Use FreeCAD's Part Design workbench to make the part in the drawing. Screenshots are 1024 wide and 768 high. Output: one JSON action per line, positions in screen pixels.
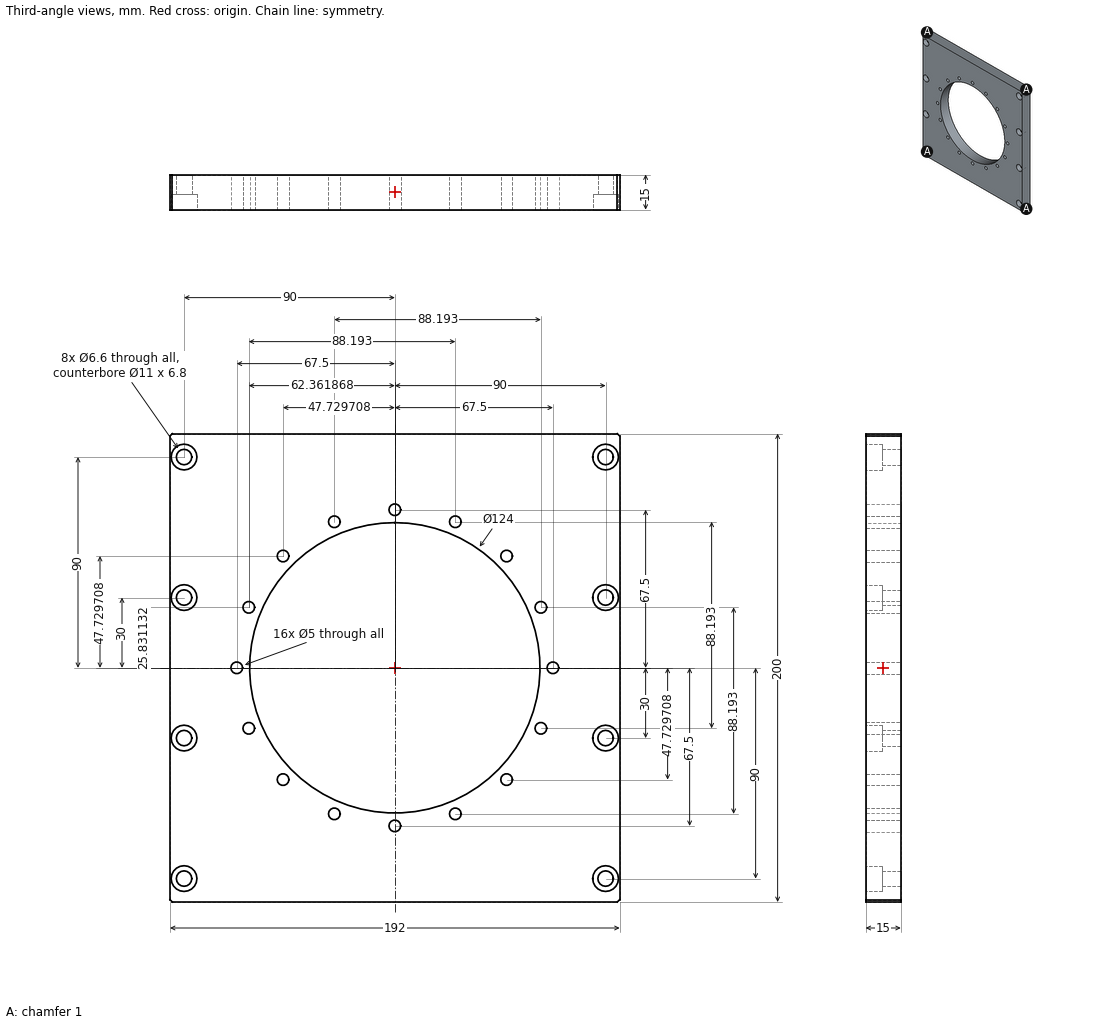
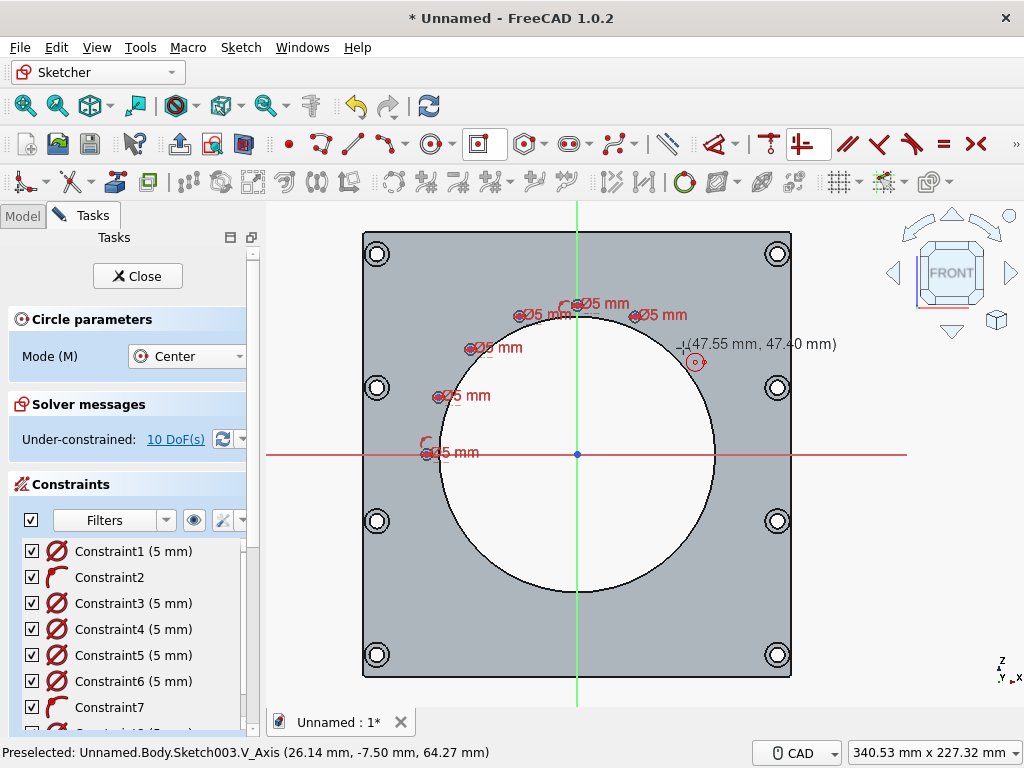
{"action": "left_click", "coordinate": [683, 348]}
{"action": "mouse_move", "coordinate": [687, 344]}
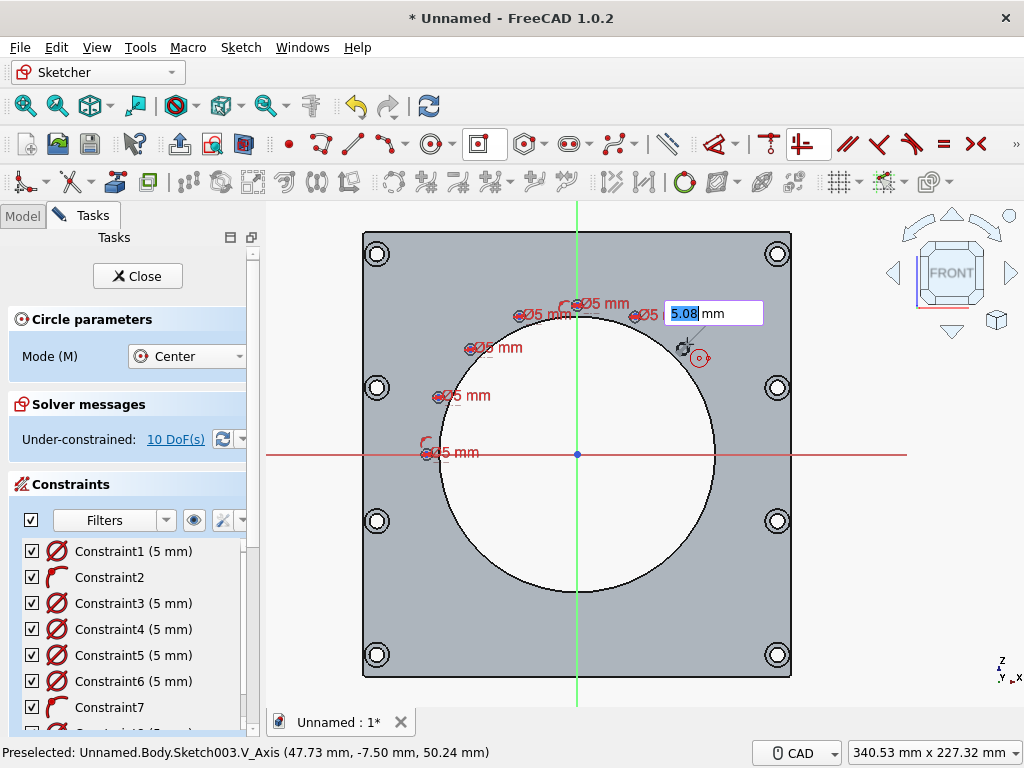
{"action": "type", "text": "5"}
{"action": "key", "text": "Return"}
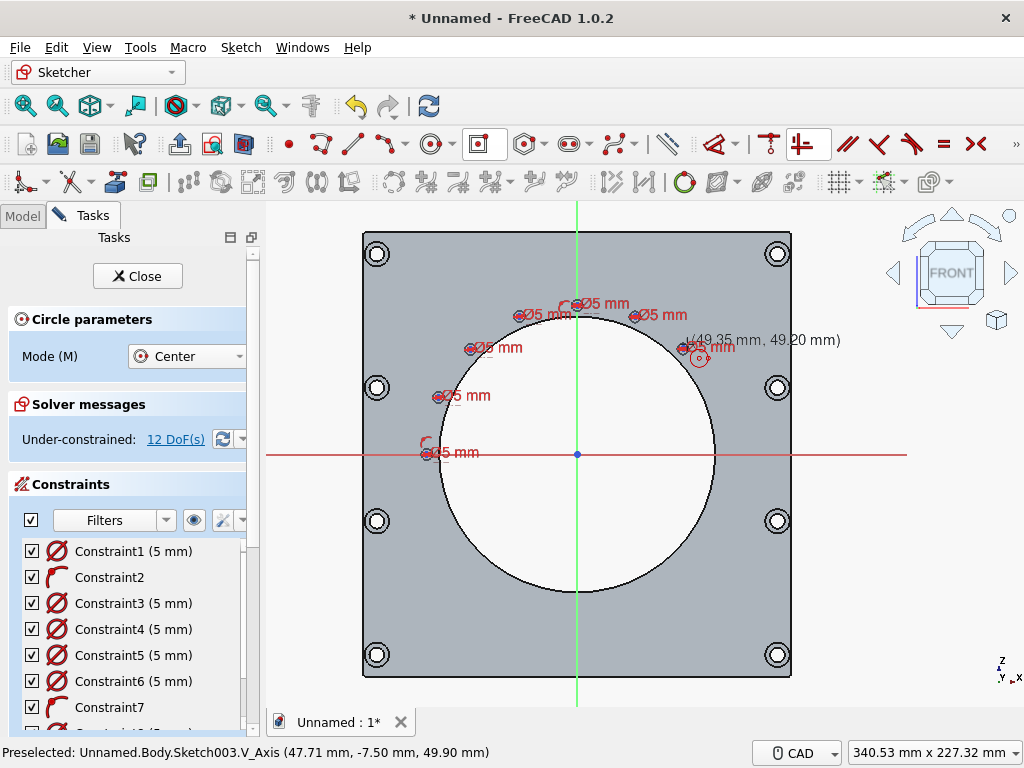
{"action": "scroll", "coordinate": [716, 397], "scroll_direction": "up", "scroll_amount": 8}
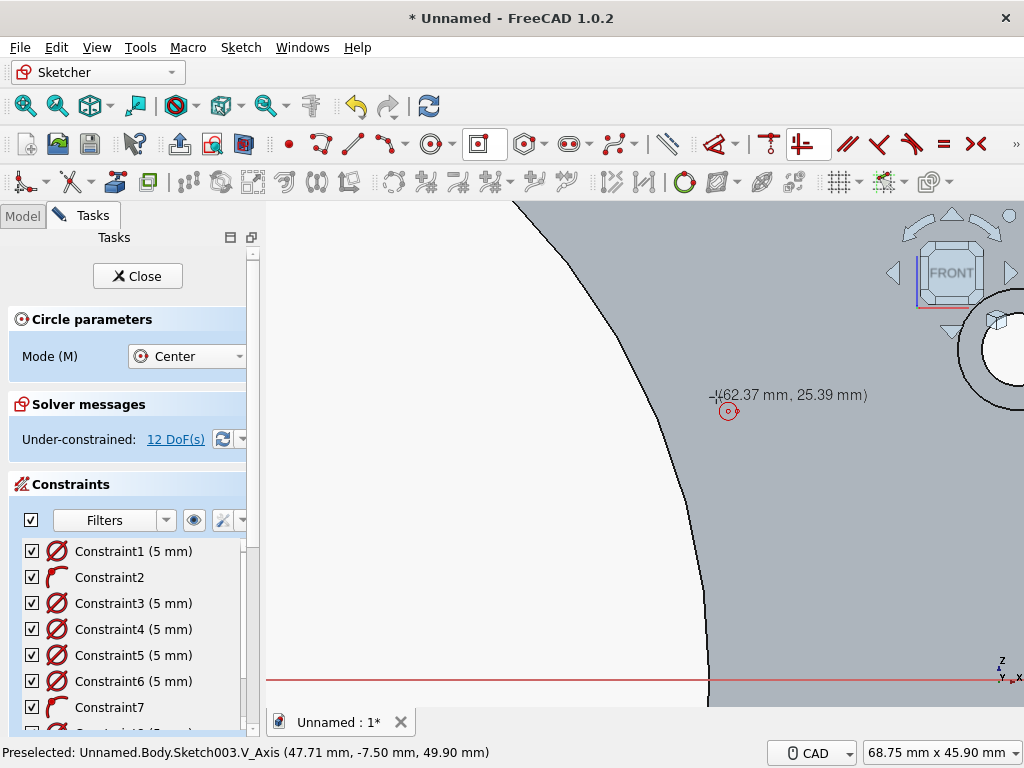
{"action": "scroll", "coordinate": [716, 397], "scroll_direction": "down", "scroll_amount": 8}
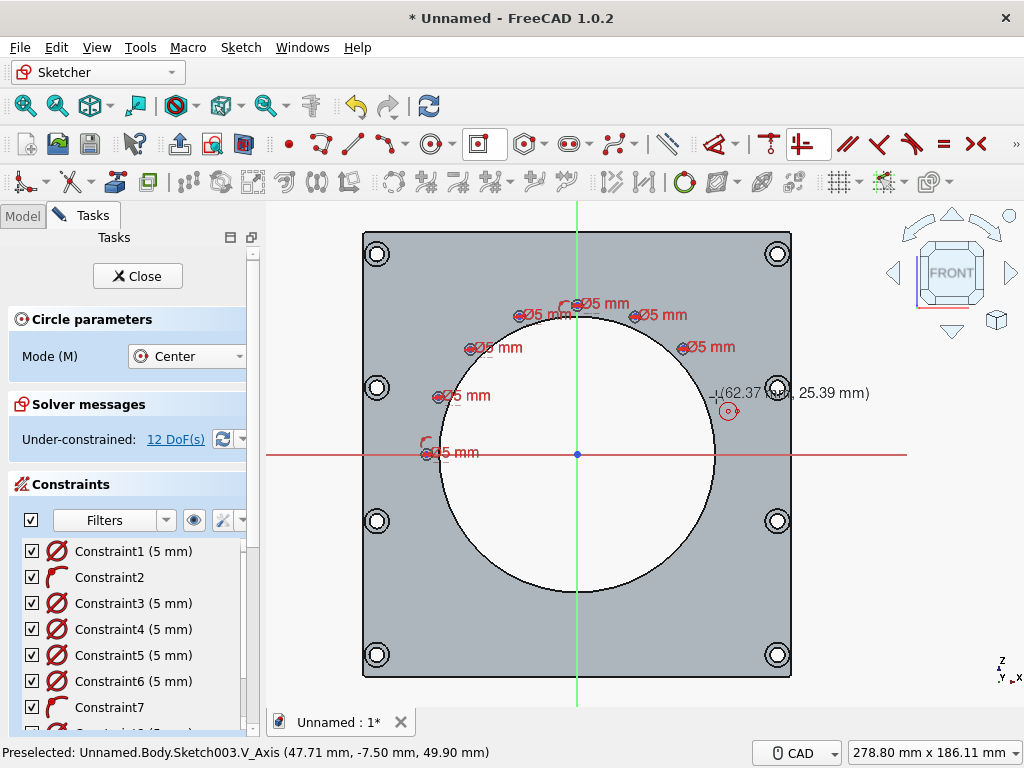
{"action": "left_click", "coordinate": [716, 397]}
{"action": "mouse_move", "coordinate": [720, 393]}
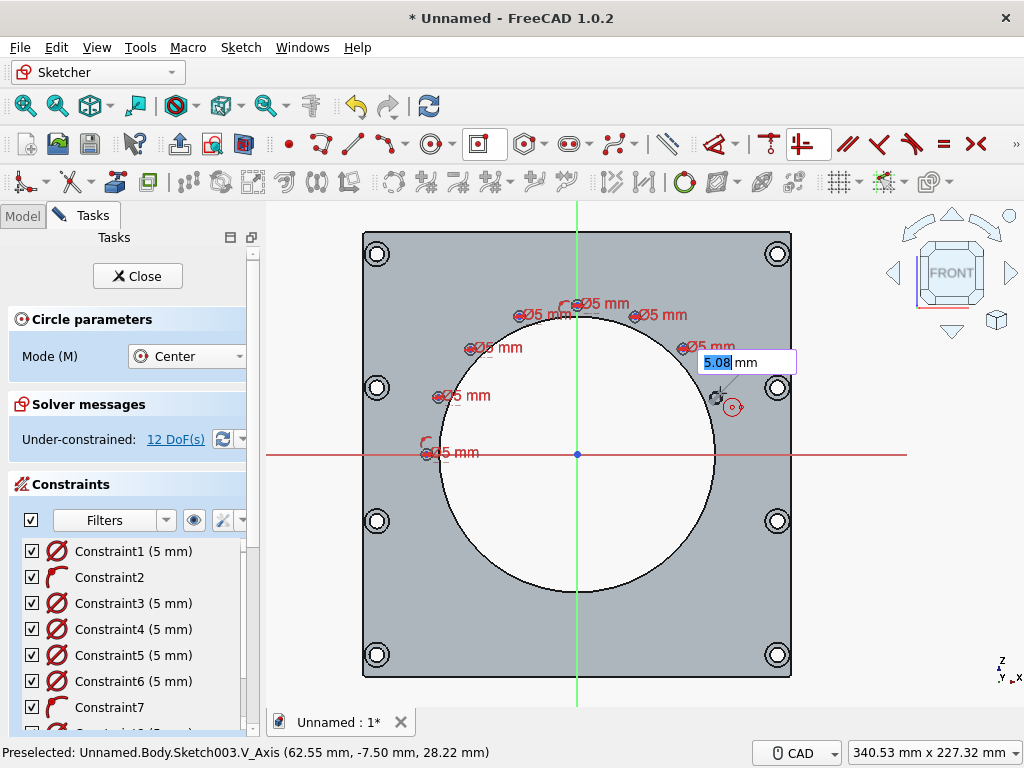
{"action": "type", "text": "5"}
{"action": "key", "text": "Return"}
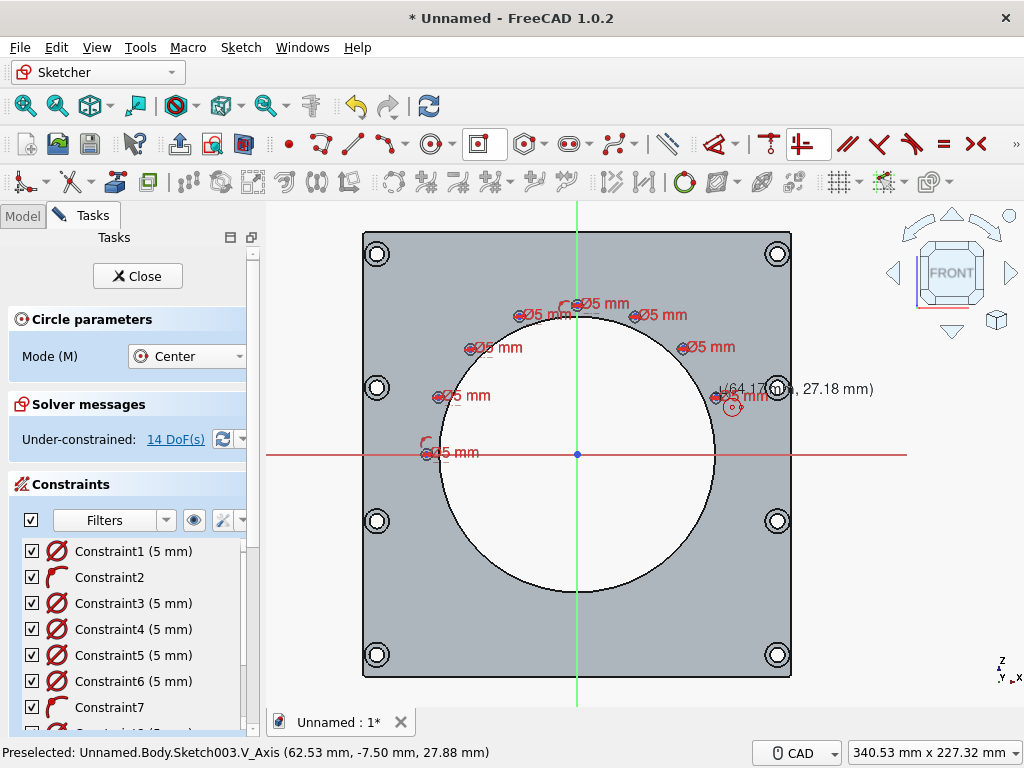
{"action": "scroll", "coordinate": [727, 455], "scroll_direction": "up", "scroll_amount": 8}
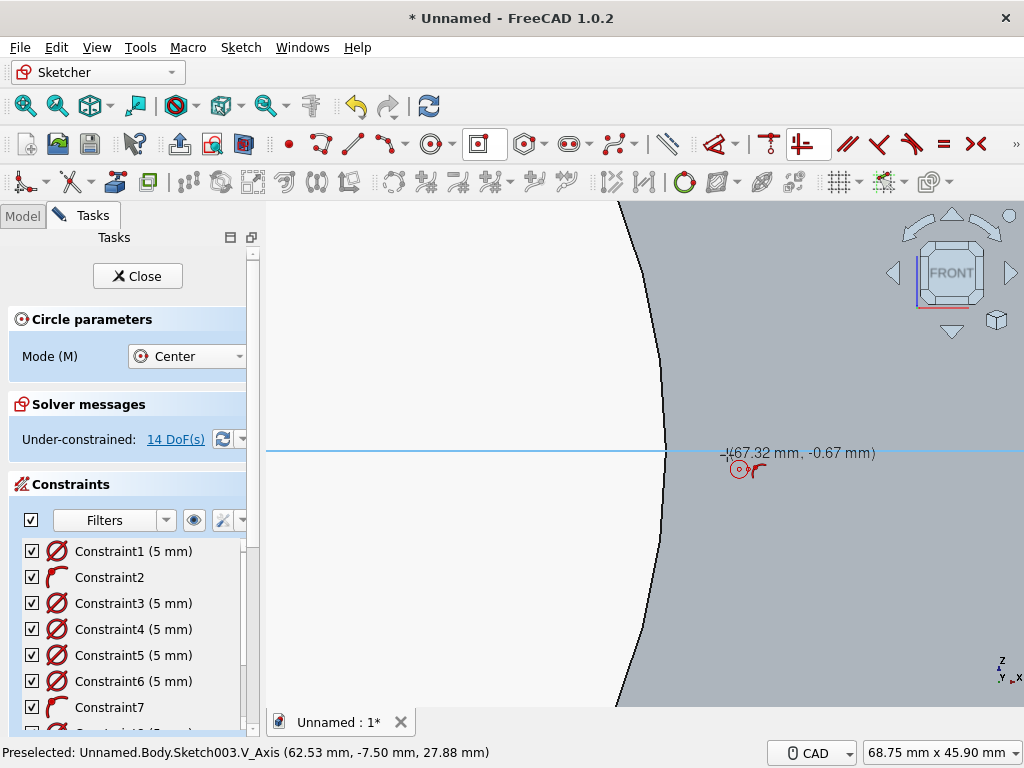
{"action": "scroll", "coordinate": [727, 455], "scroll_direction": "down", "scroll_amount": 8}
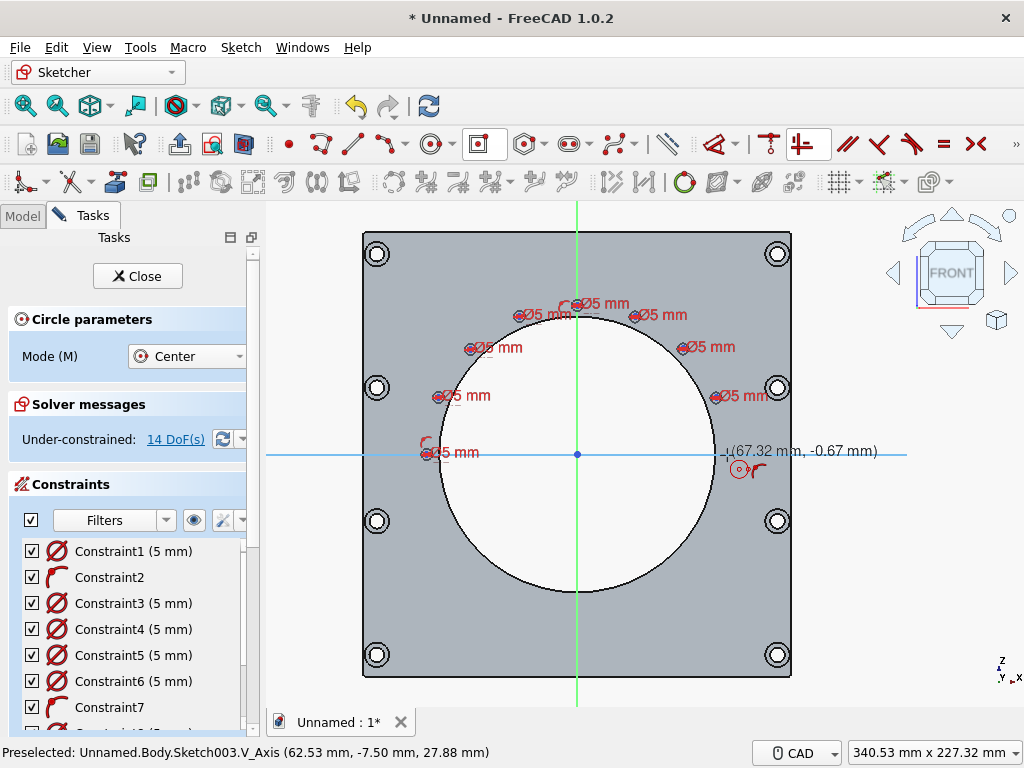
{"action": "left_click", "coordinate": [727, 455]}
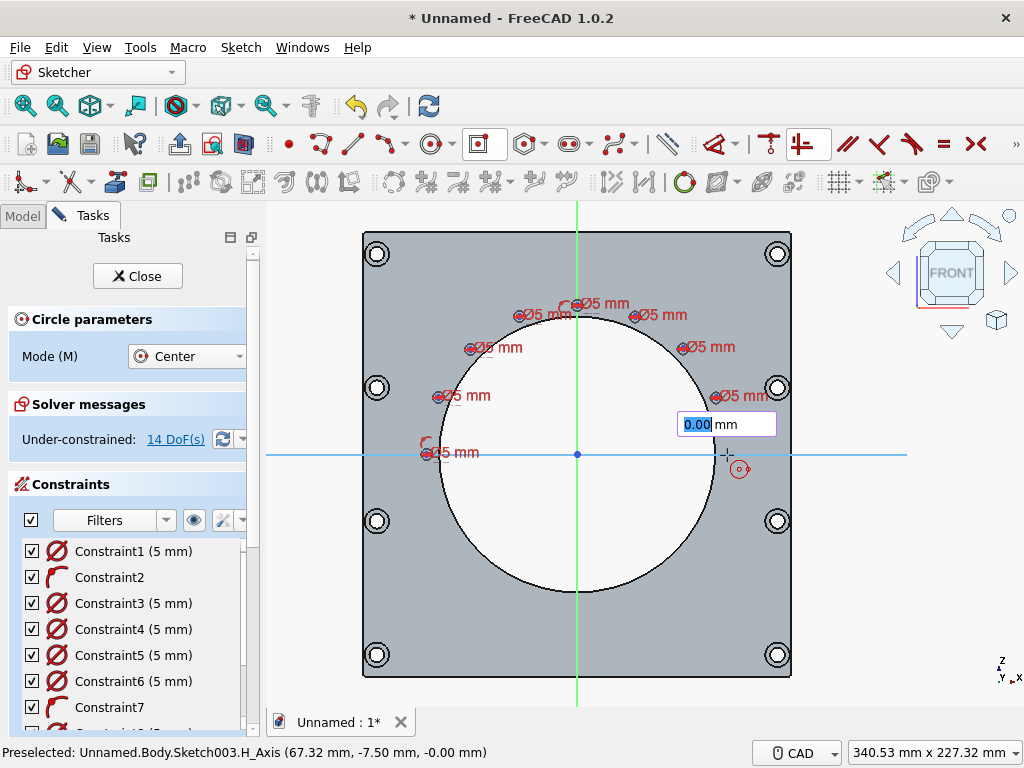
{"action": "scroll", "coordinate": [726, 460], "scroll_direction": "up", "scroll_amount": 6}
{"action": "mouse_move", "coordinate": [723, 458]}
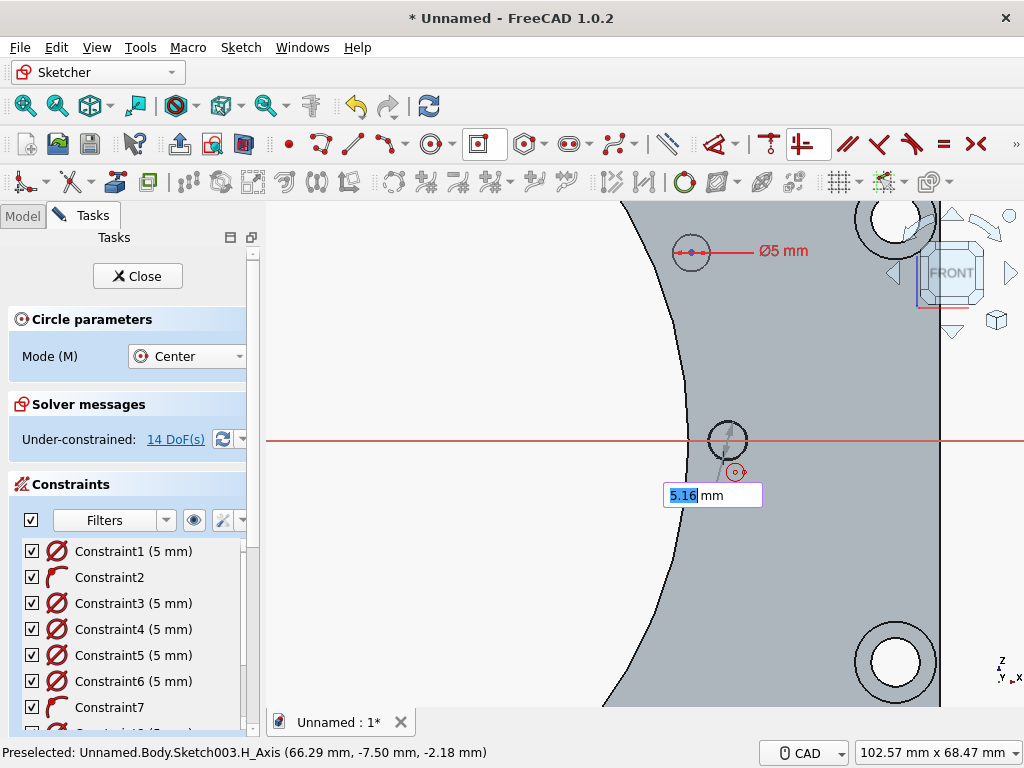
{"action": "type", "text": "5"}
{"action": "key", "text": "Return"}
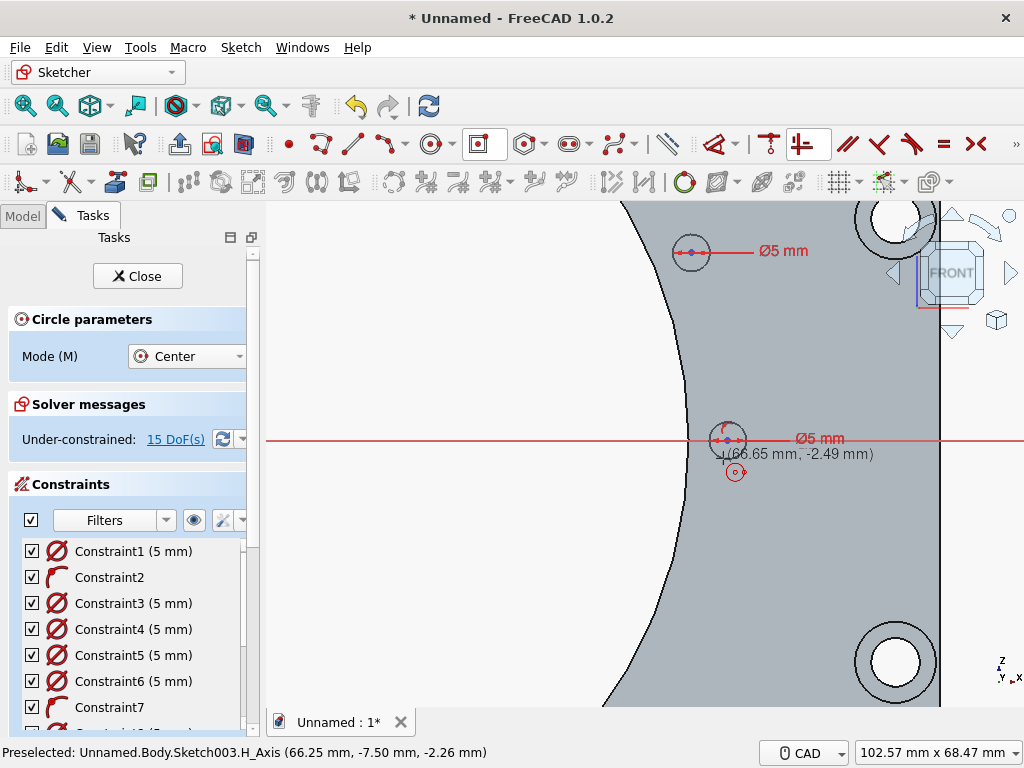
{"action": "scroll", "coordinate": [691, 631], "scroll_direction": "up", "scroll_amount": 2}